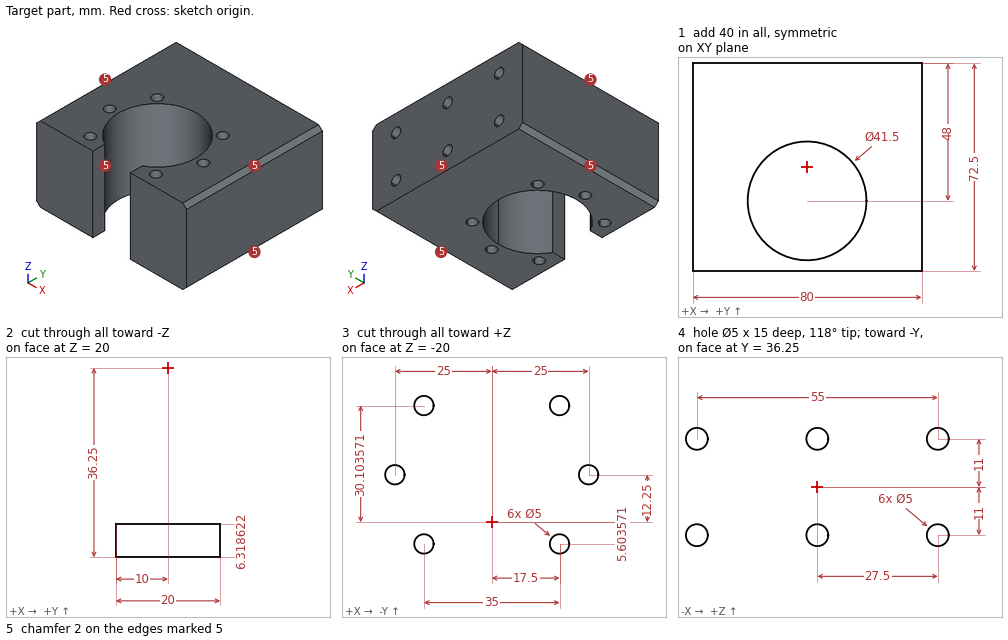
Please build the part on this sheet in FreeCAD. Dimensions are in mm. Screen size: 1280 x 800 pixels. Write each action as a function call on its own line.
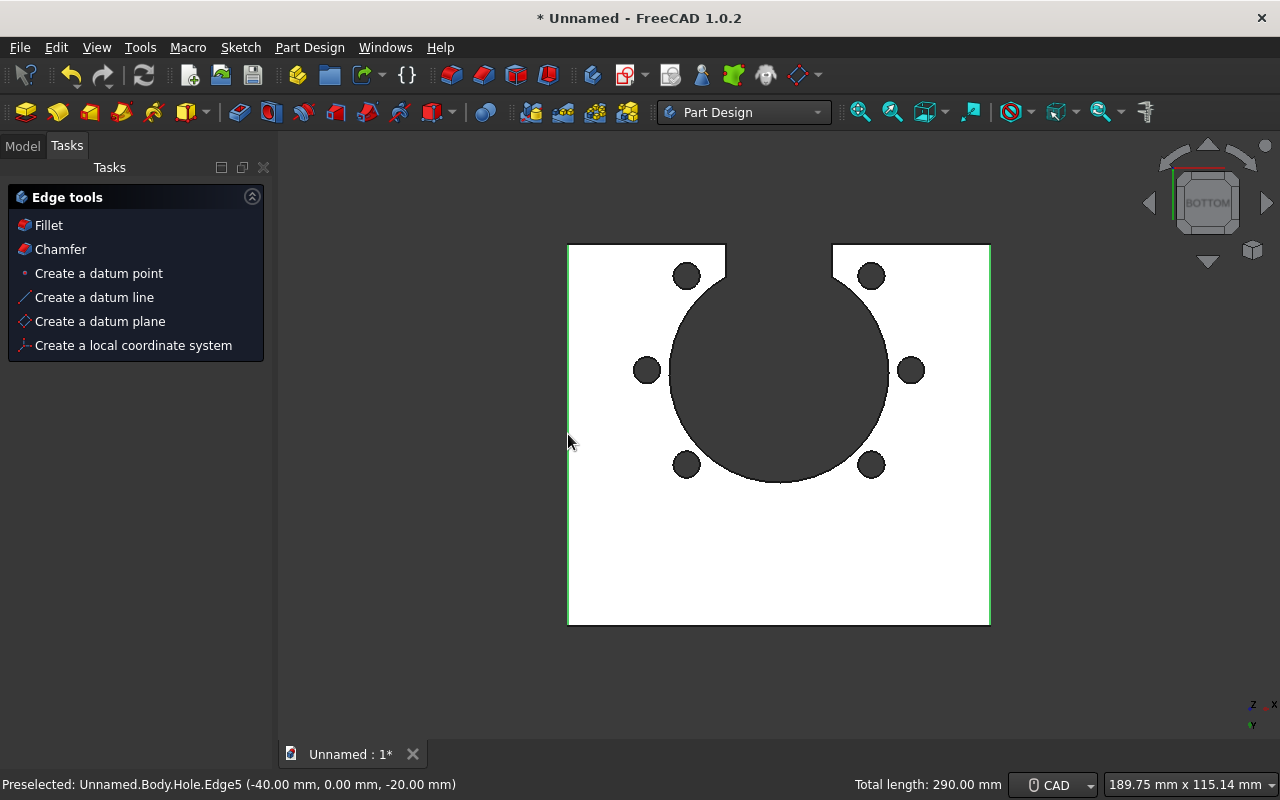
click(484, 76)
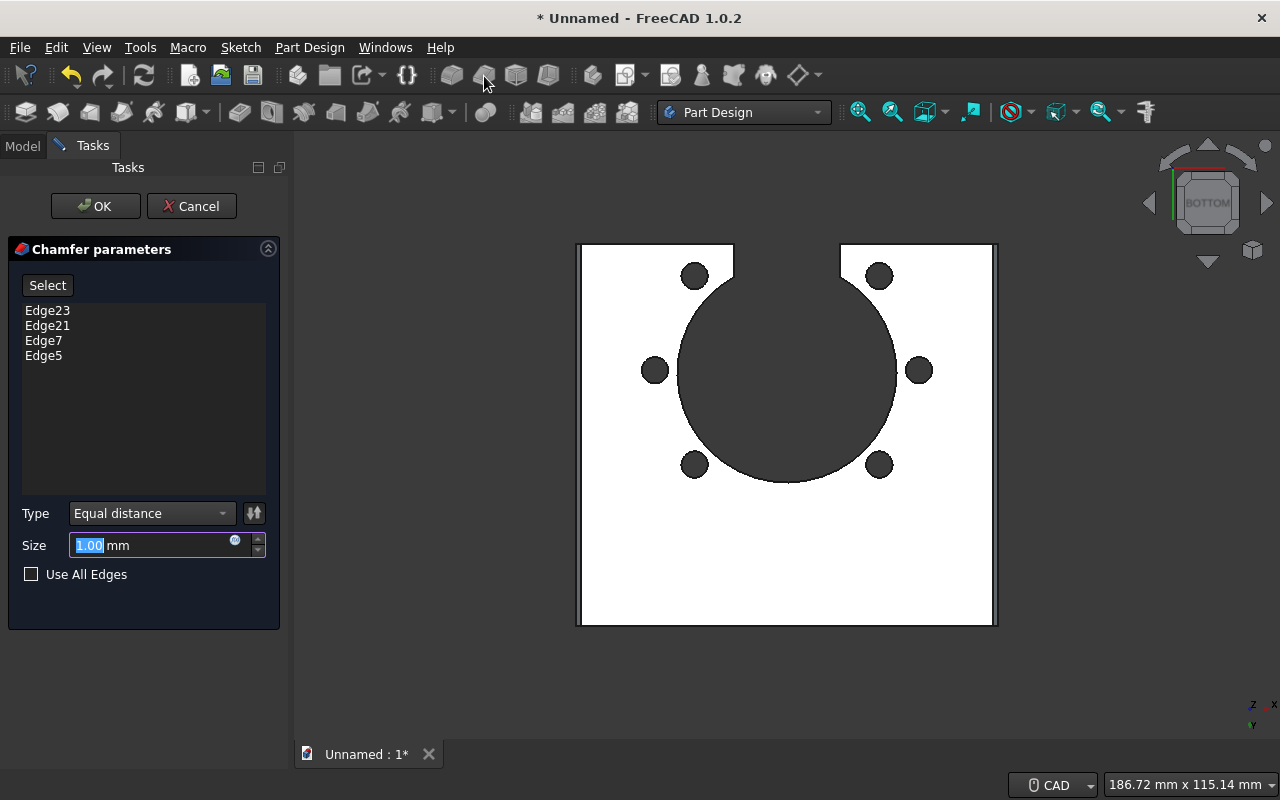
text(2)
key(Tab)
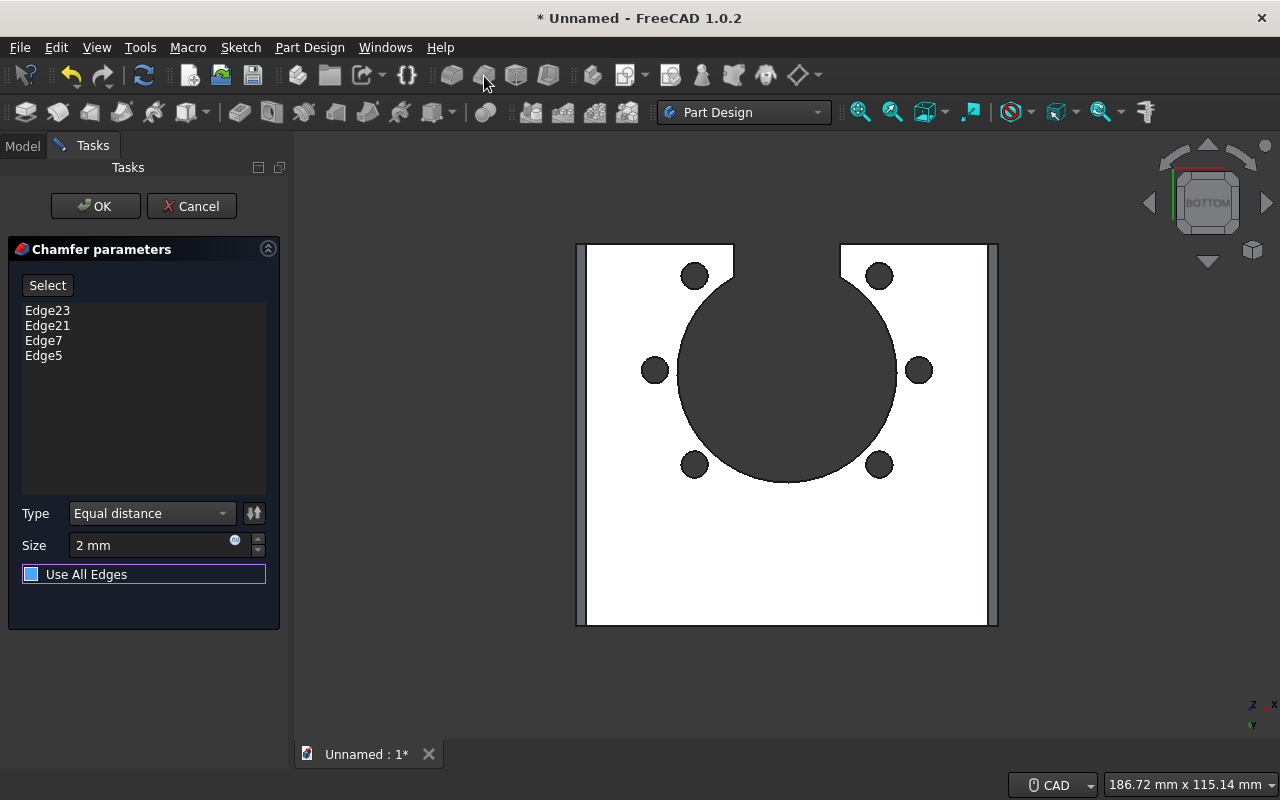
click(96, 206)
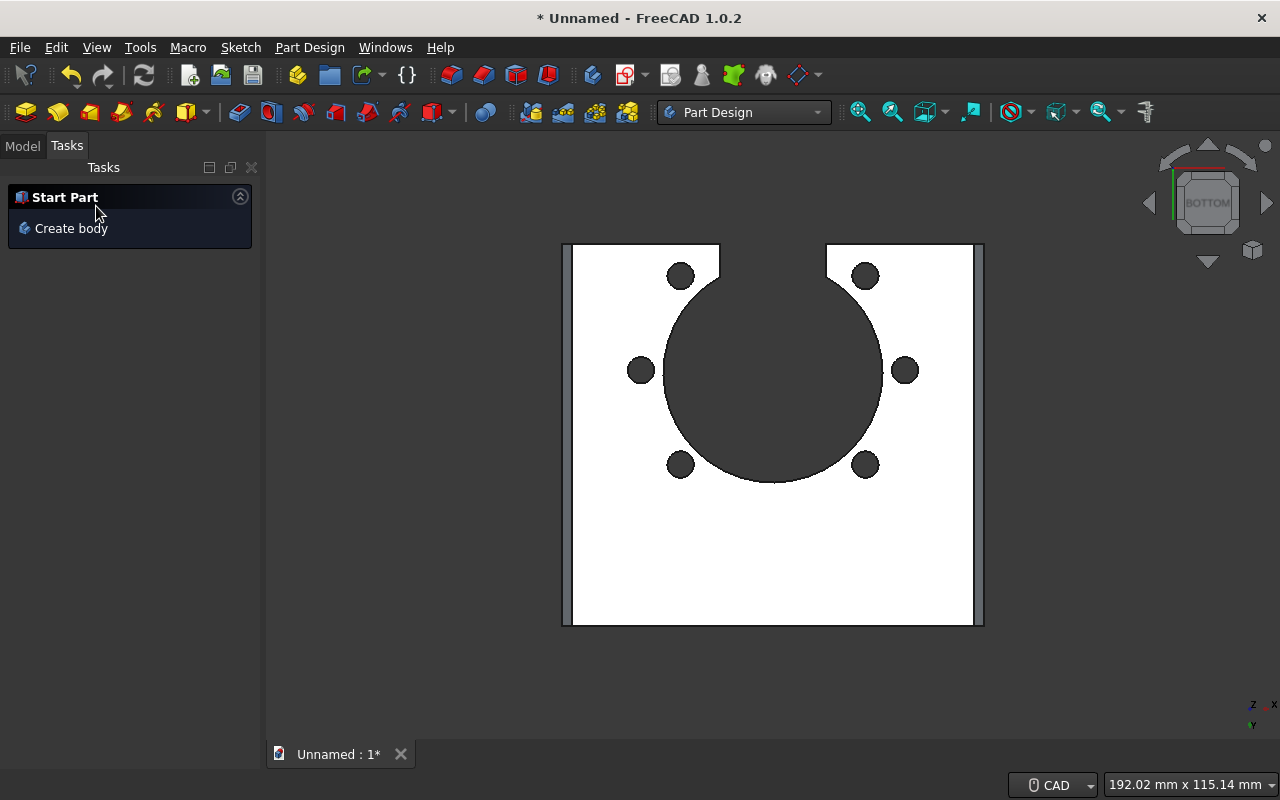
key(0)